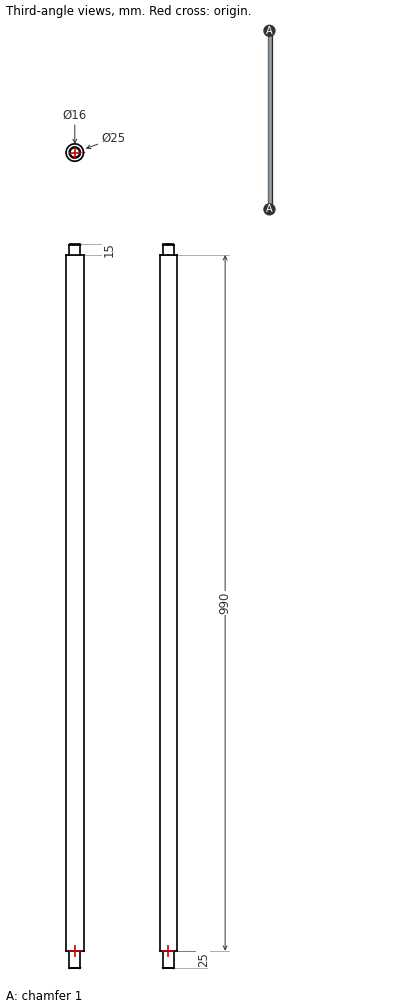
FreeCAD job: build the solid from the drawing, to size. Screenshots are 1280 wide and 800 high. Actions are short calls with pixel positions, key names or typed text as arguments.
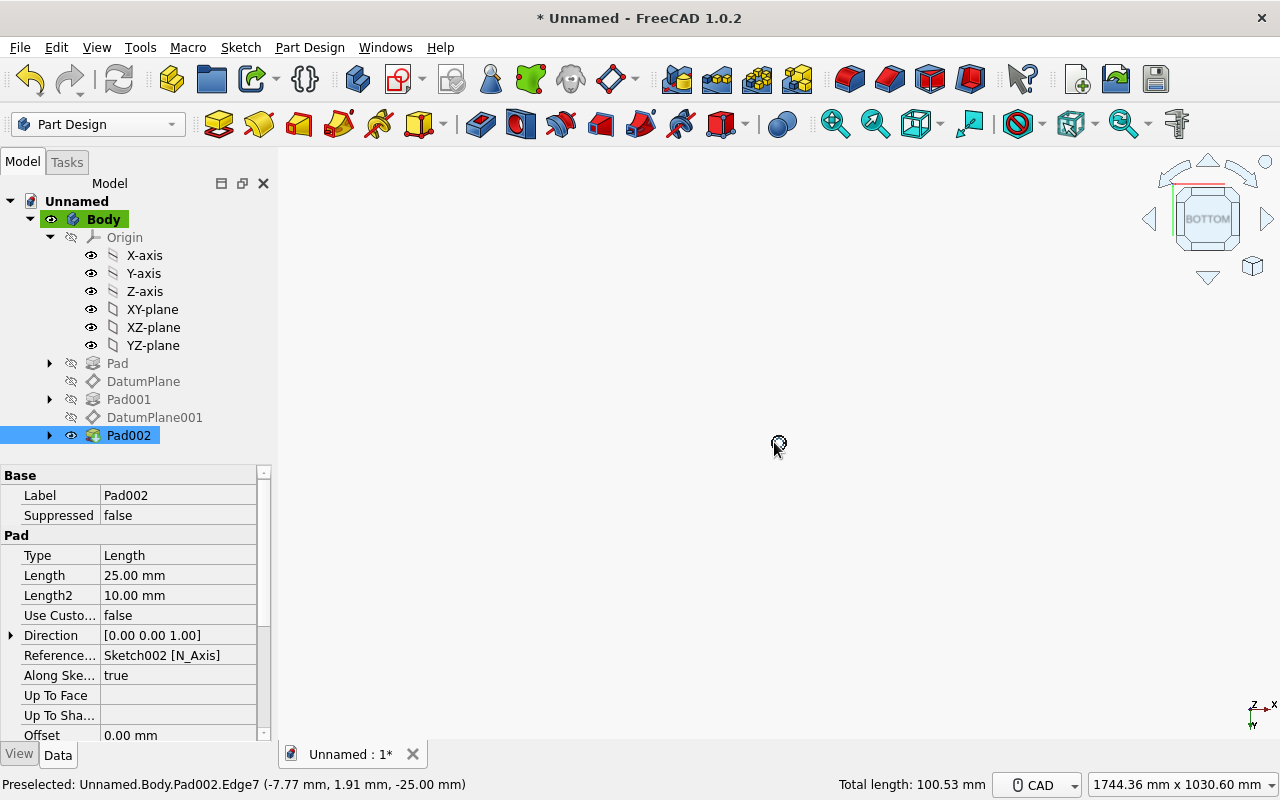
click(890, 80)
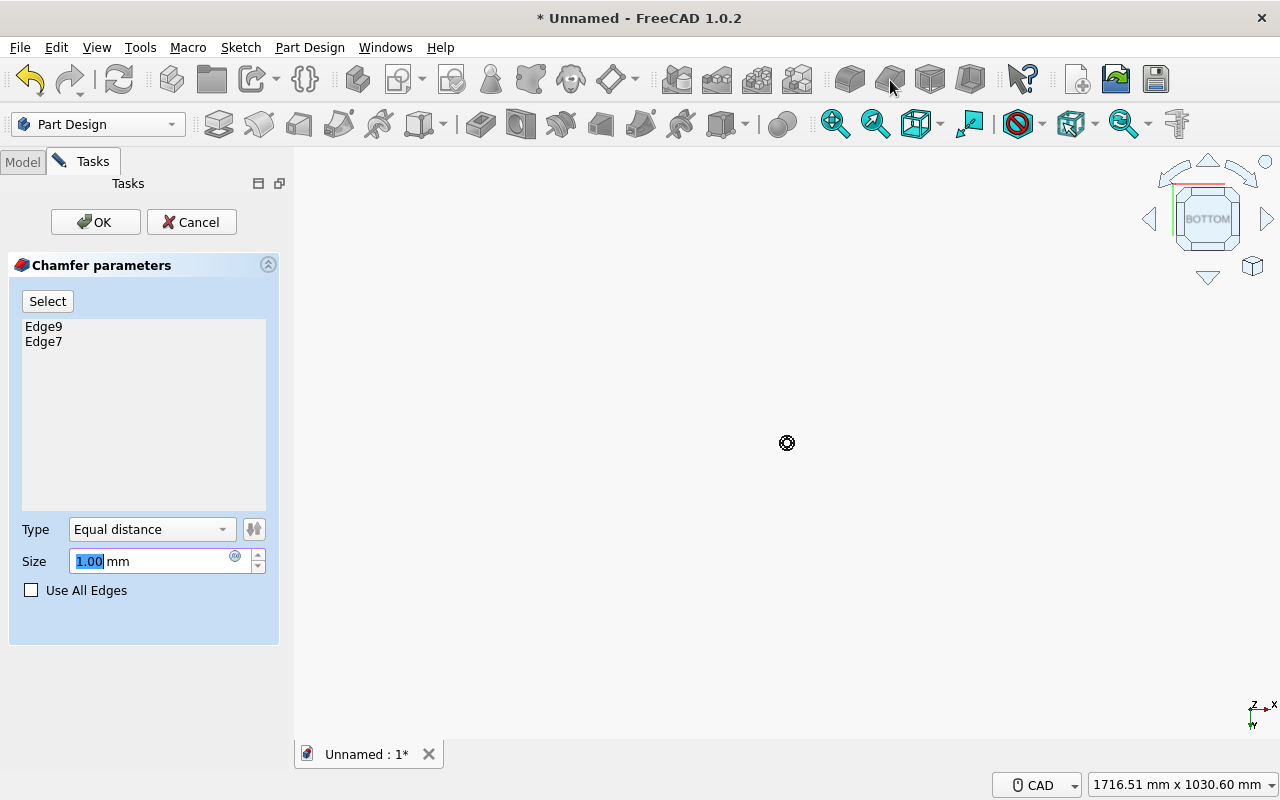
text(1)
key(Tab)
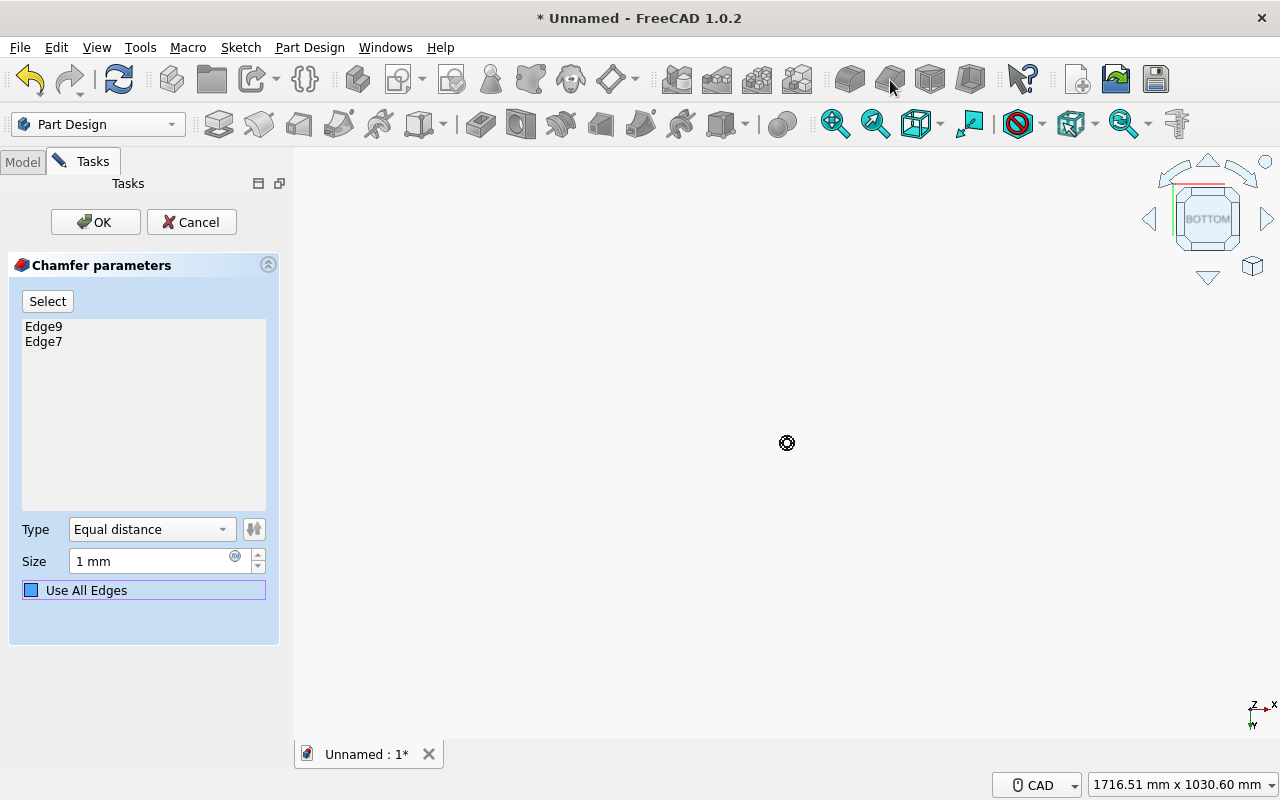
click(96, 222)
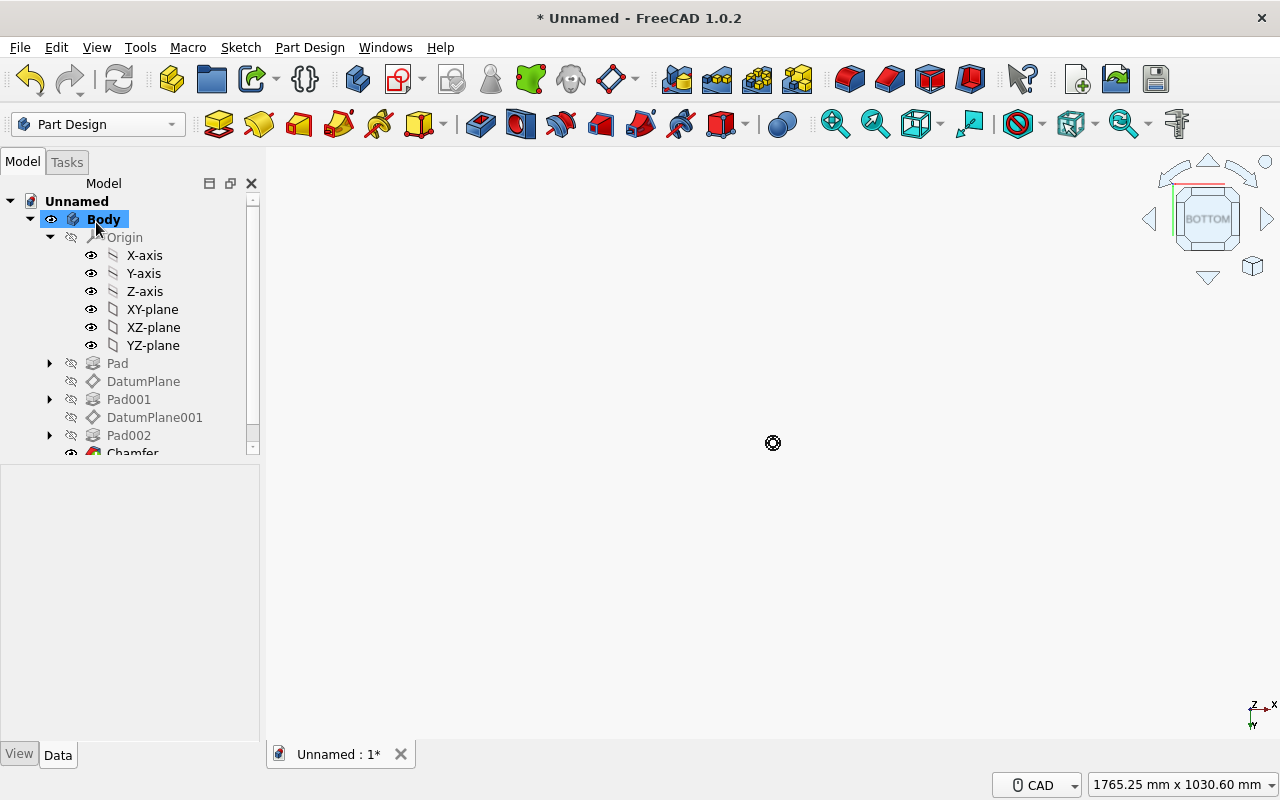
key(0)